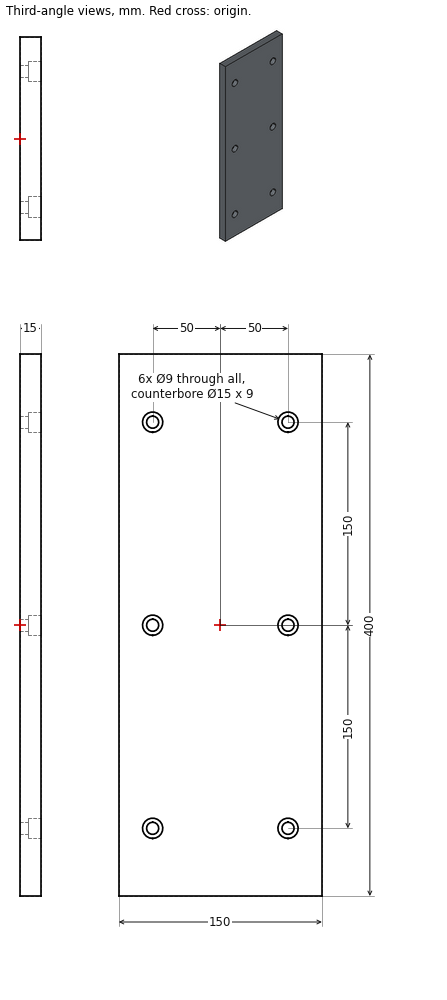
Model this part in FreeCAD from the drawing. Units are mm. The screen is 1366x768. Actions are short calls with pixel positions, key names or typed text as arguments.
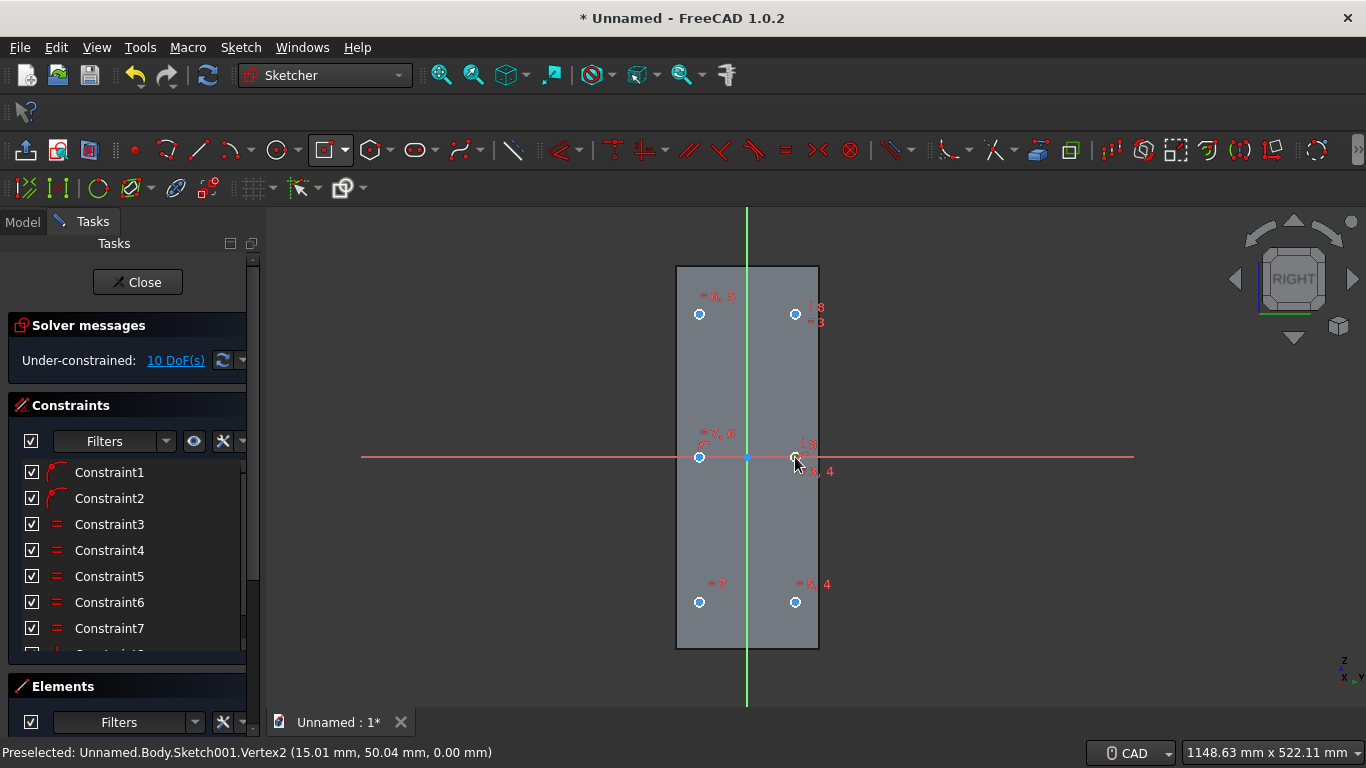
click(795, 602)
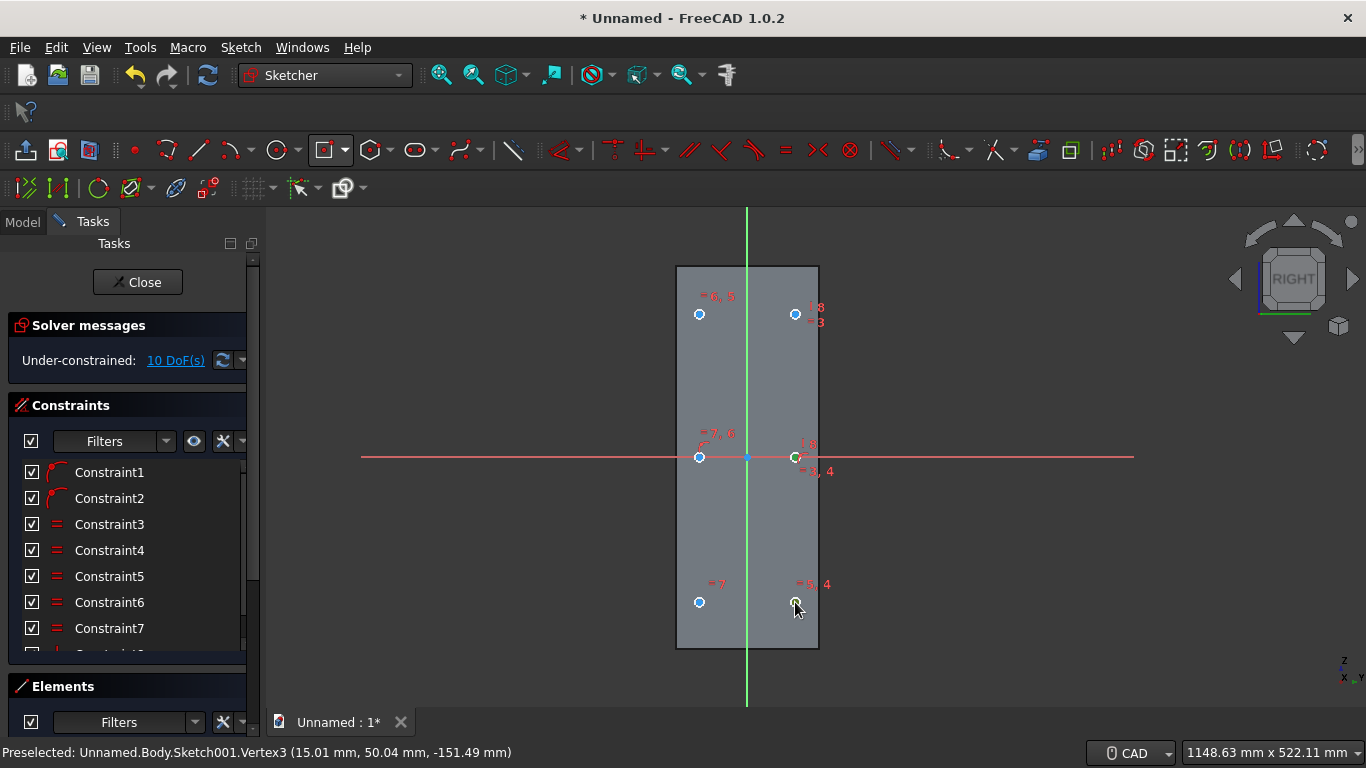
key(v)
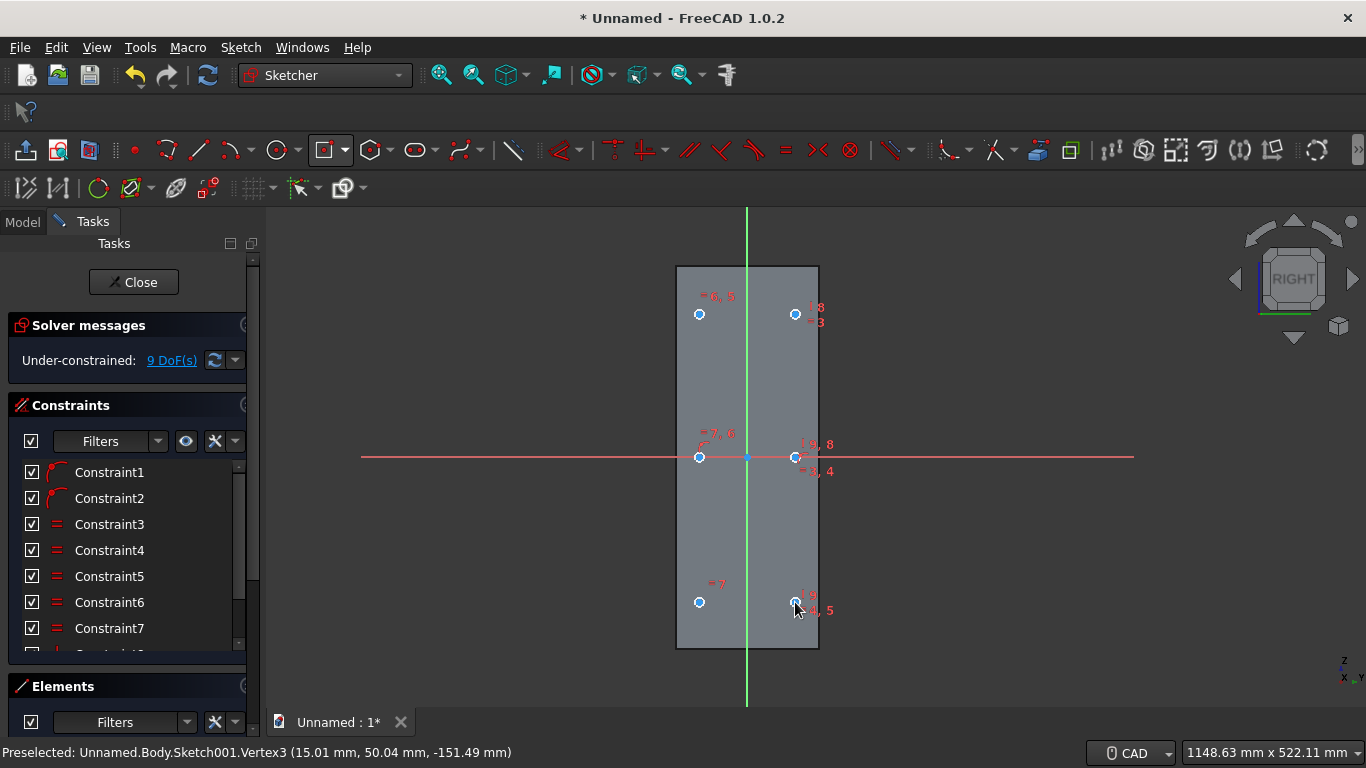
click(795, 314)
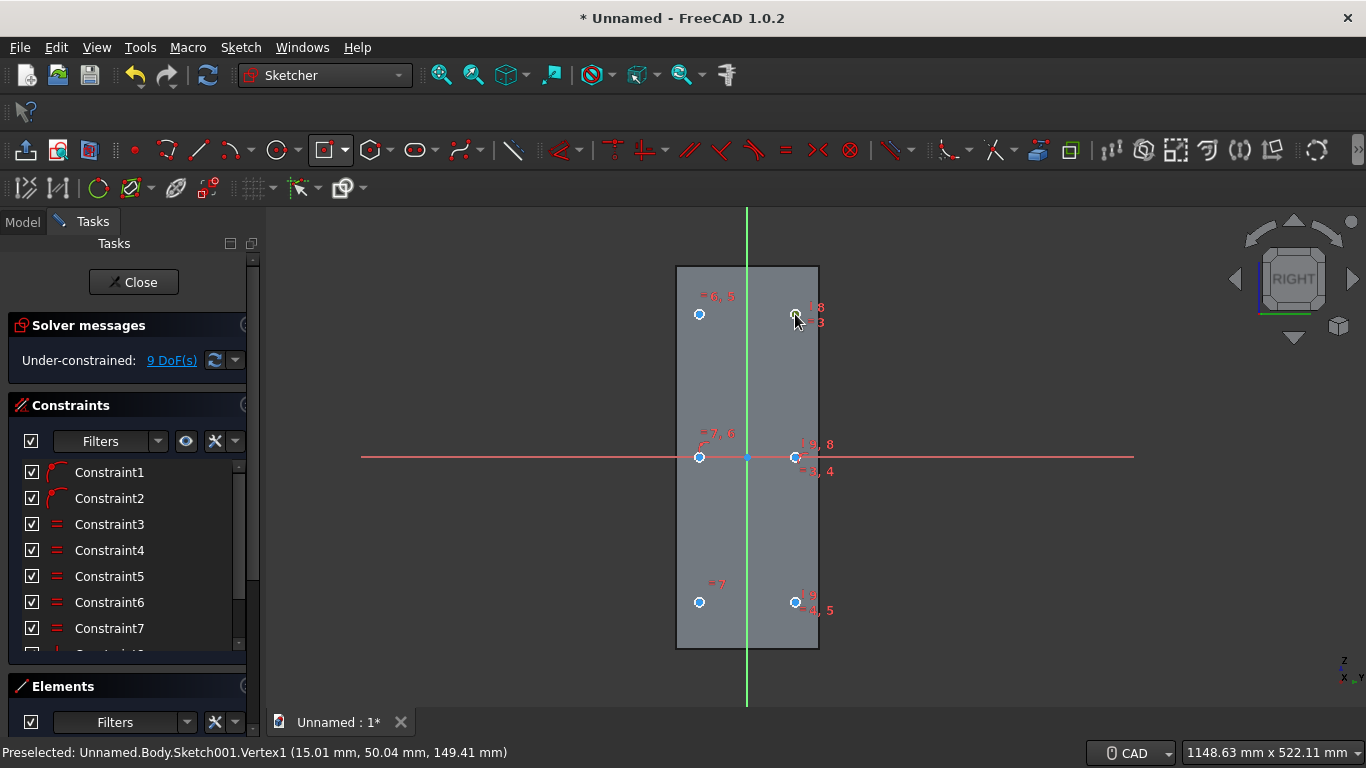
click(699, 314)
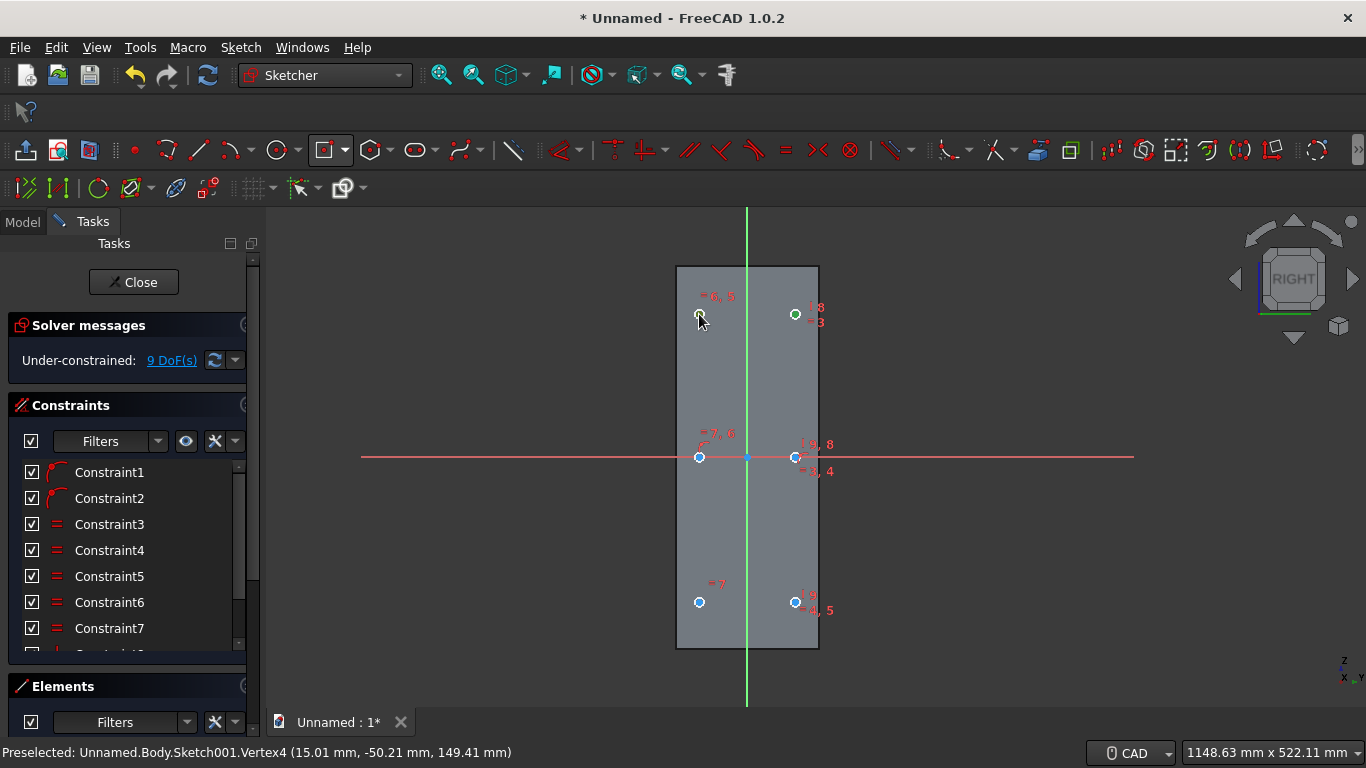
key(h)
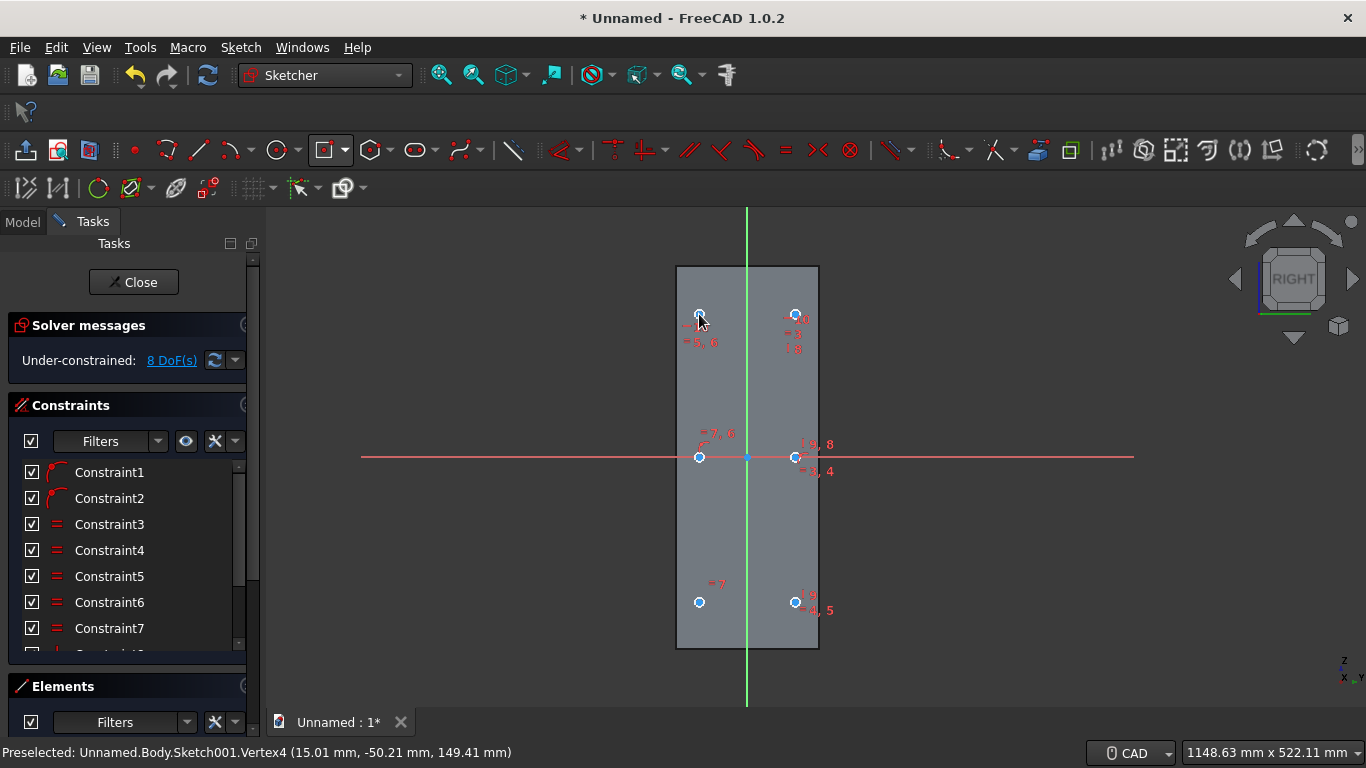
click(699, 314)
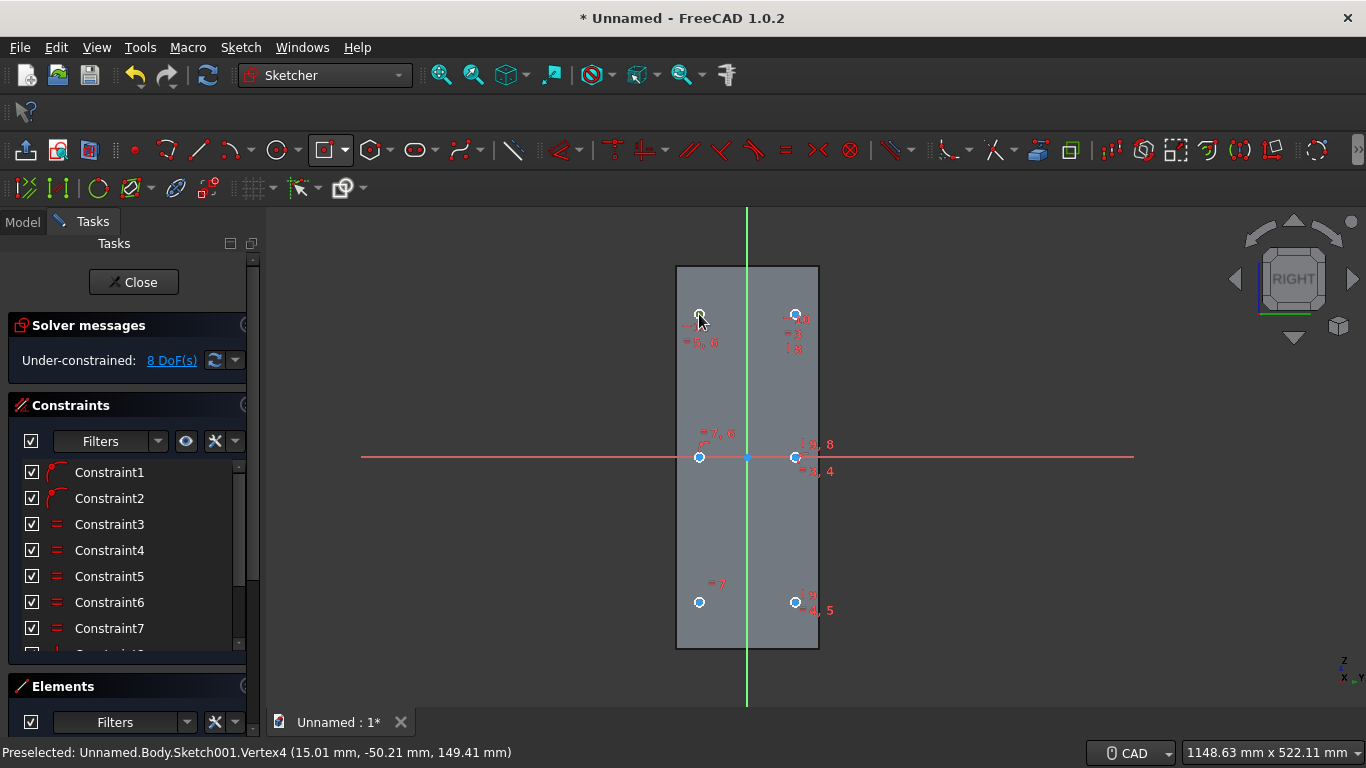
click(699, 457)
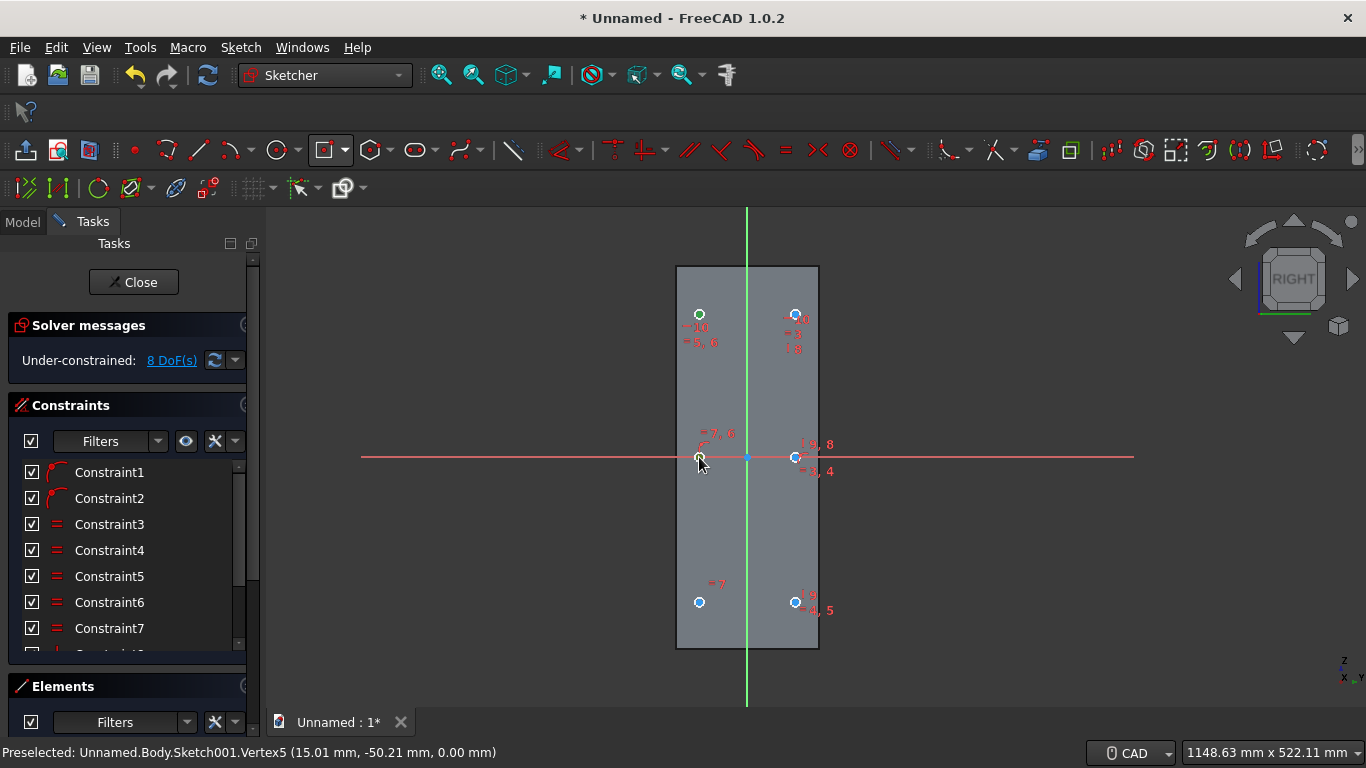
key(v)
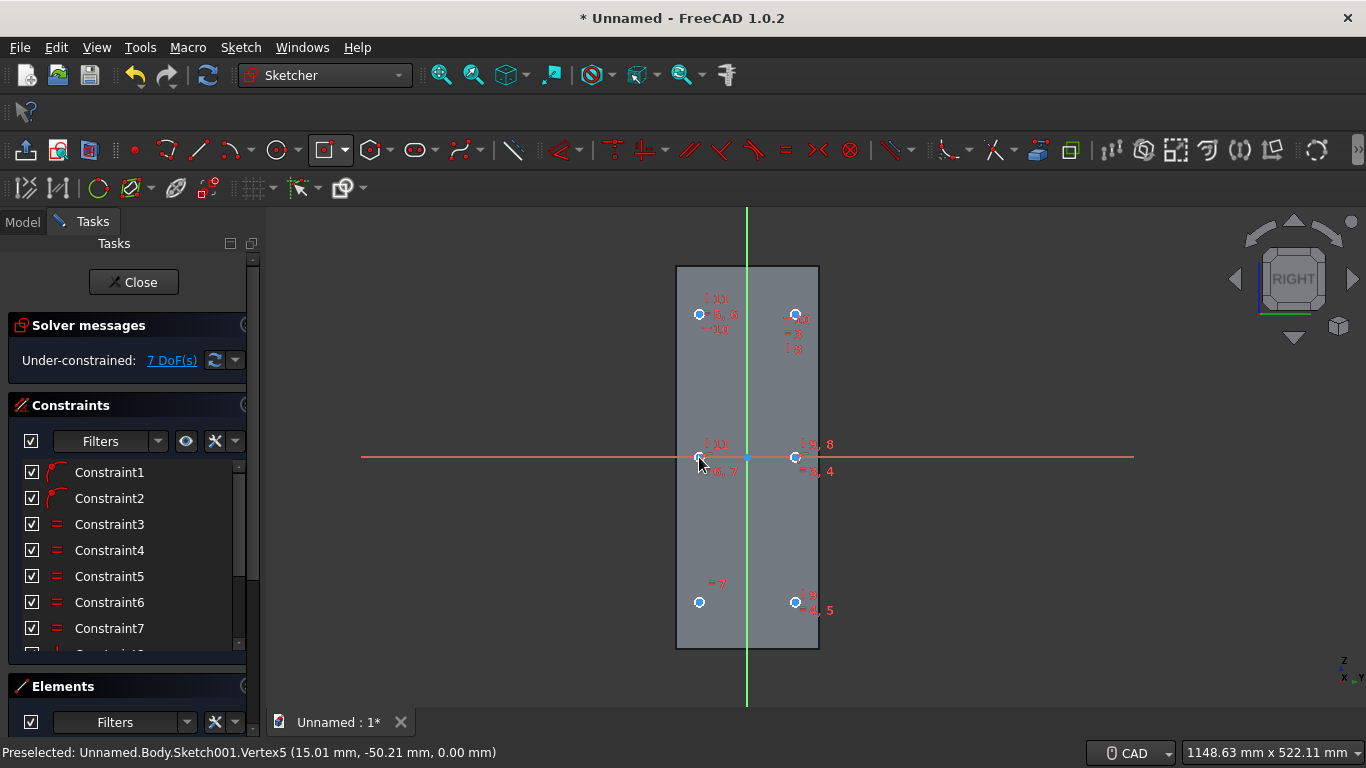
click(699, 457)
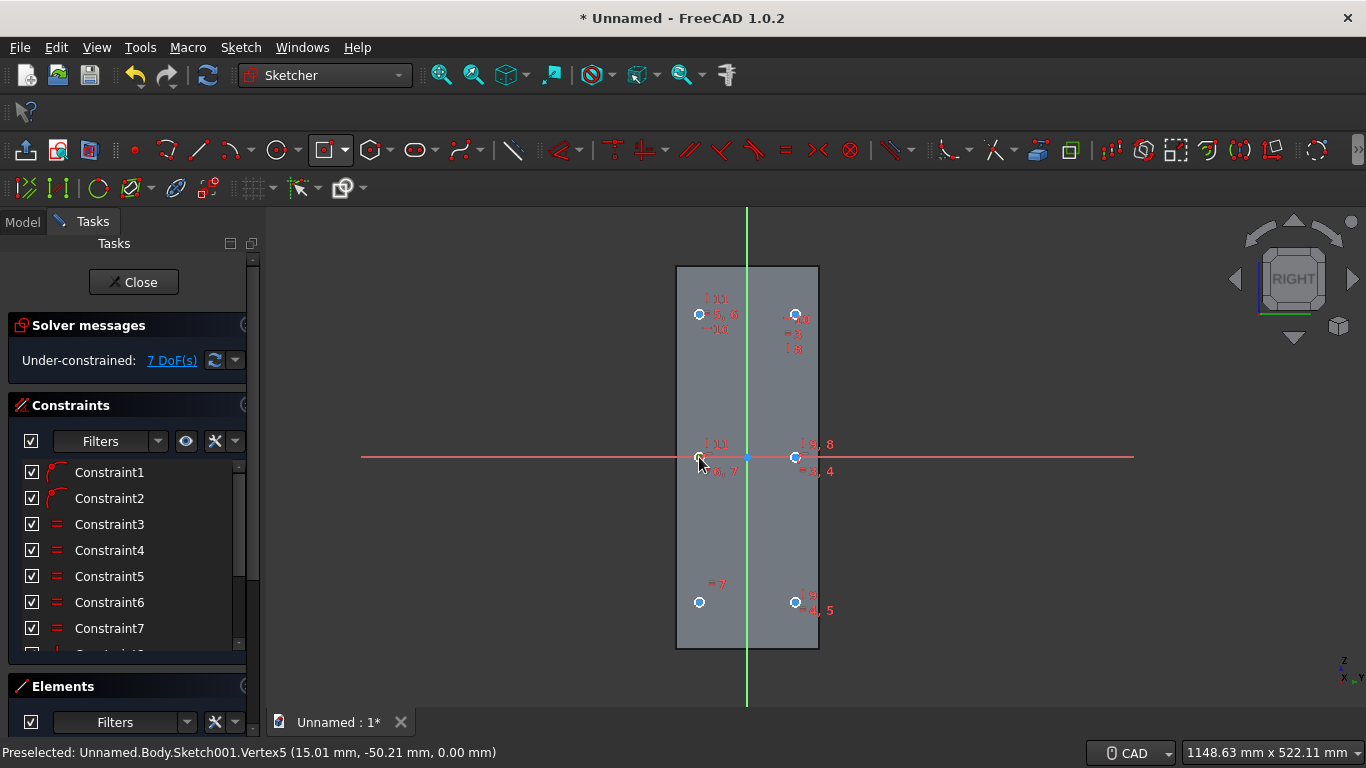
click(699, 602)